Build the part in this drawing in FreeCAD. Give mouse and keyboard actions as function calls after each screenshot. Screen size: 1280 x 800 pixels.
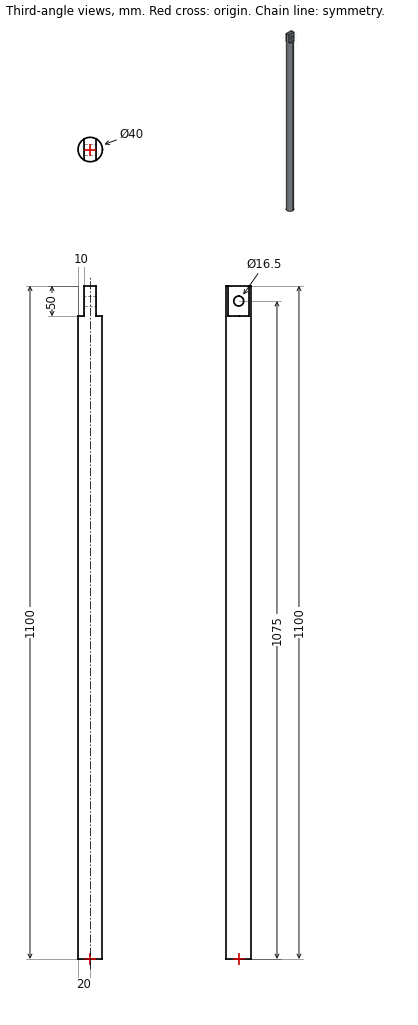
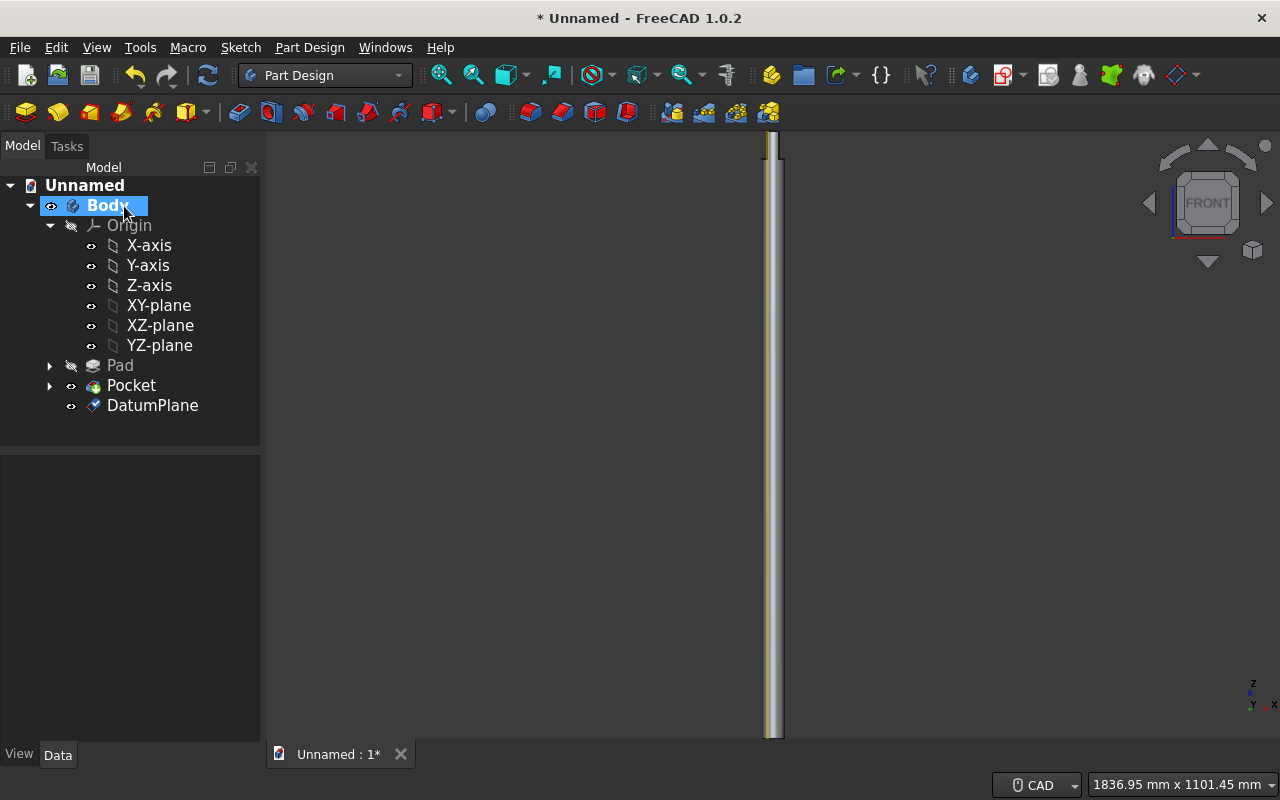
click(116, 406)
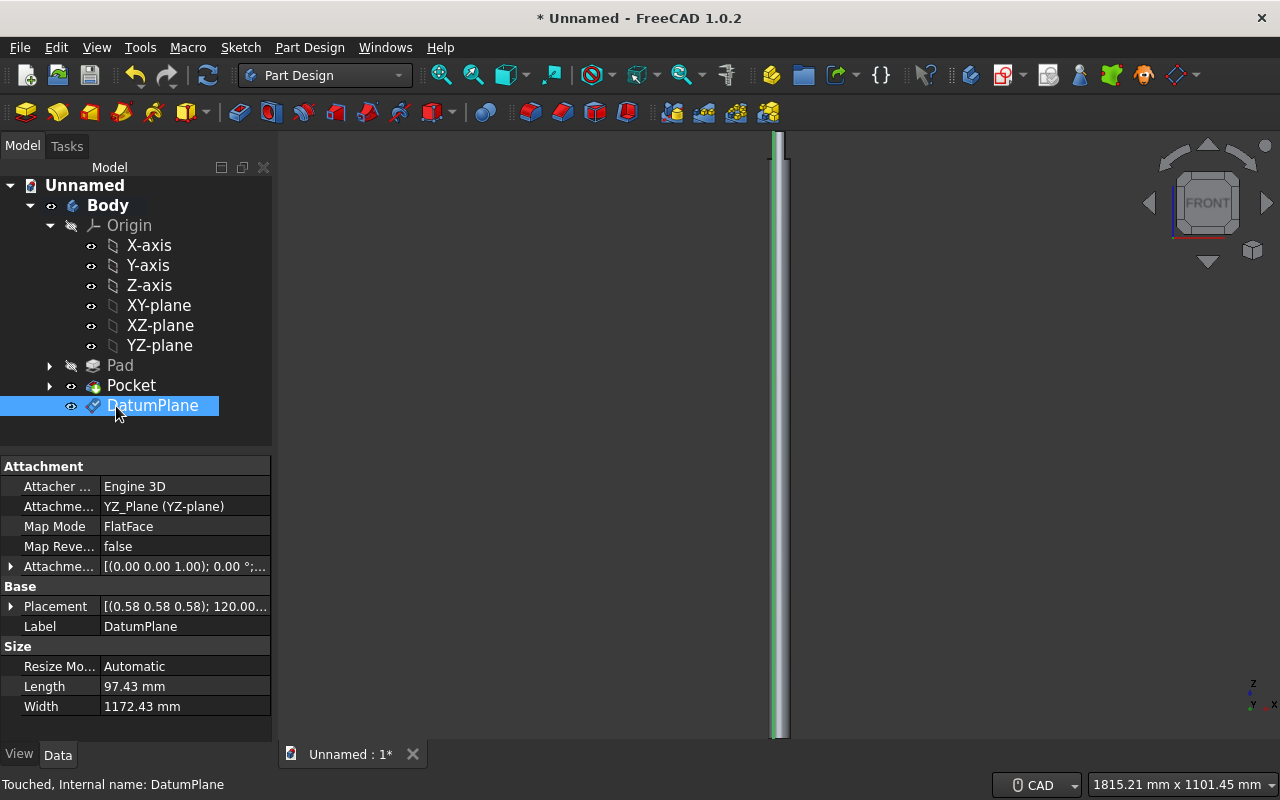
click(1004, 76)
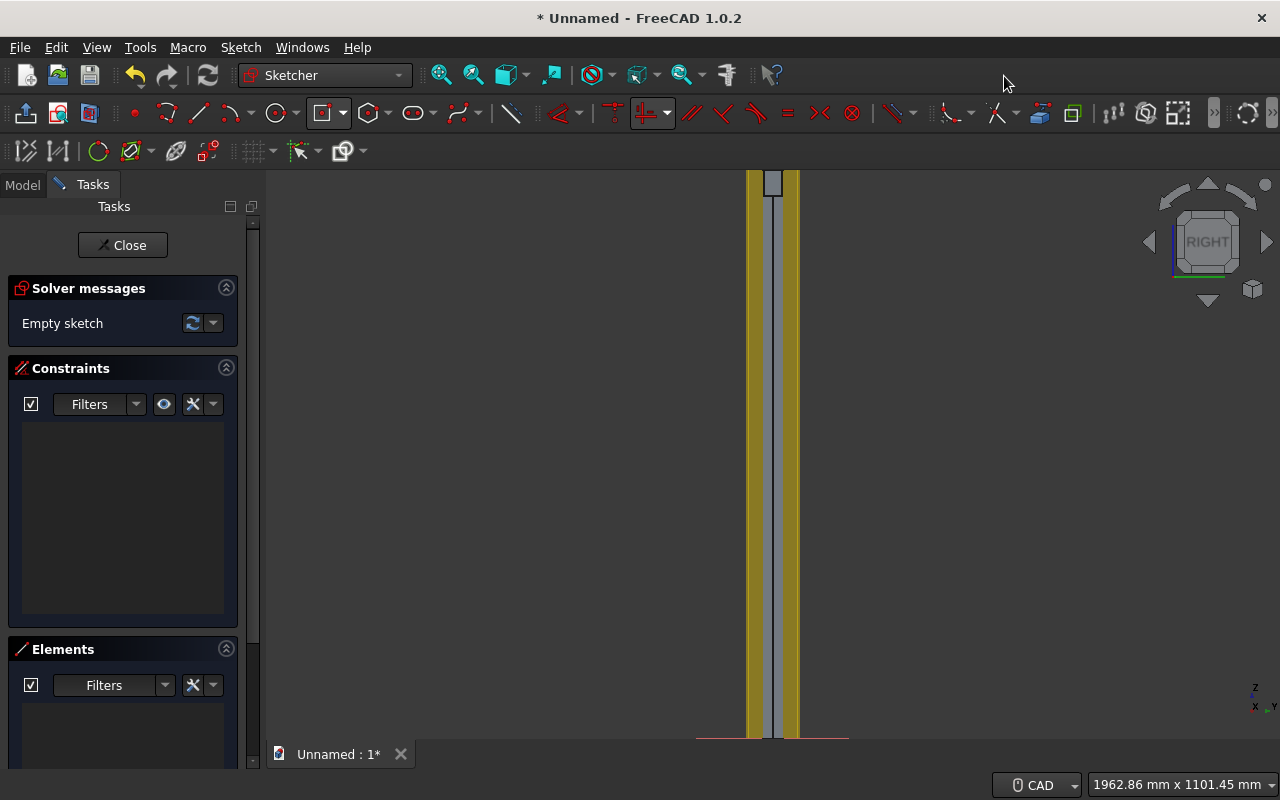
click(90, 114)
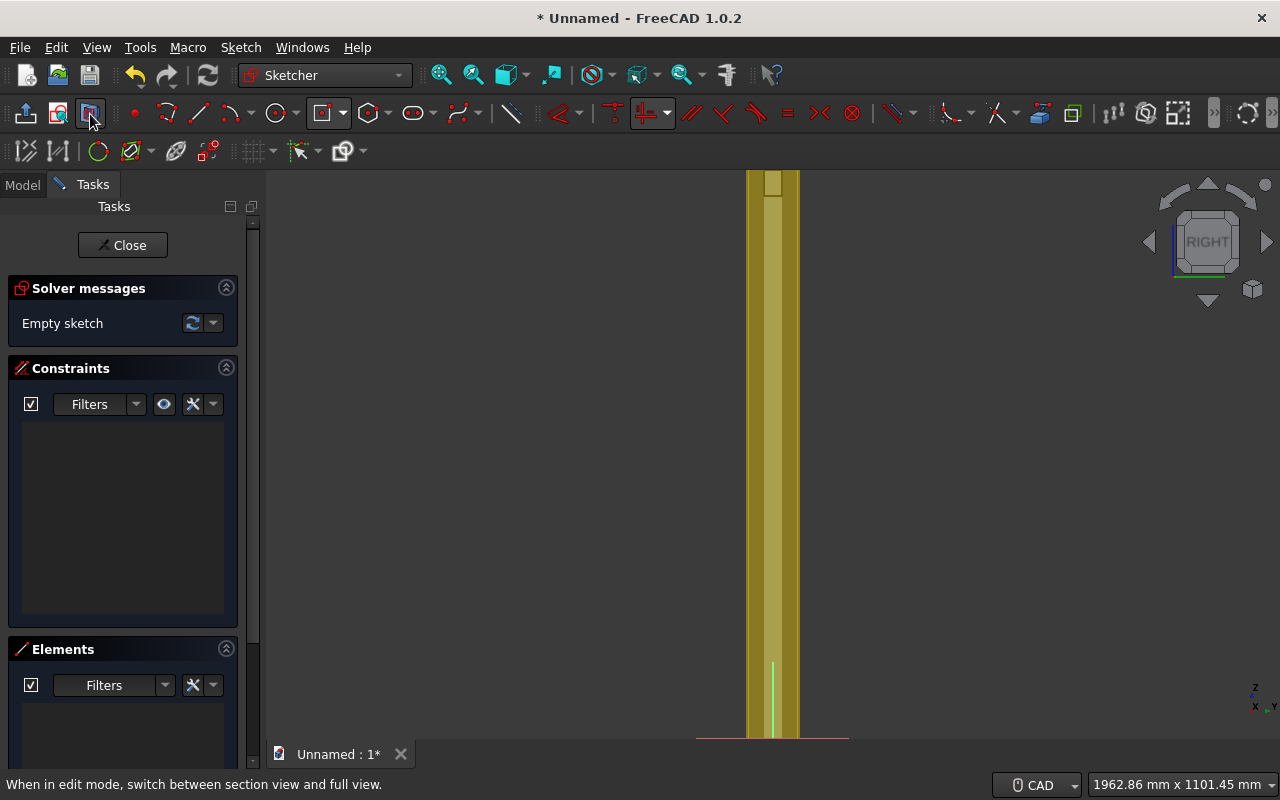
scroll(704, 454, down, 5)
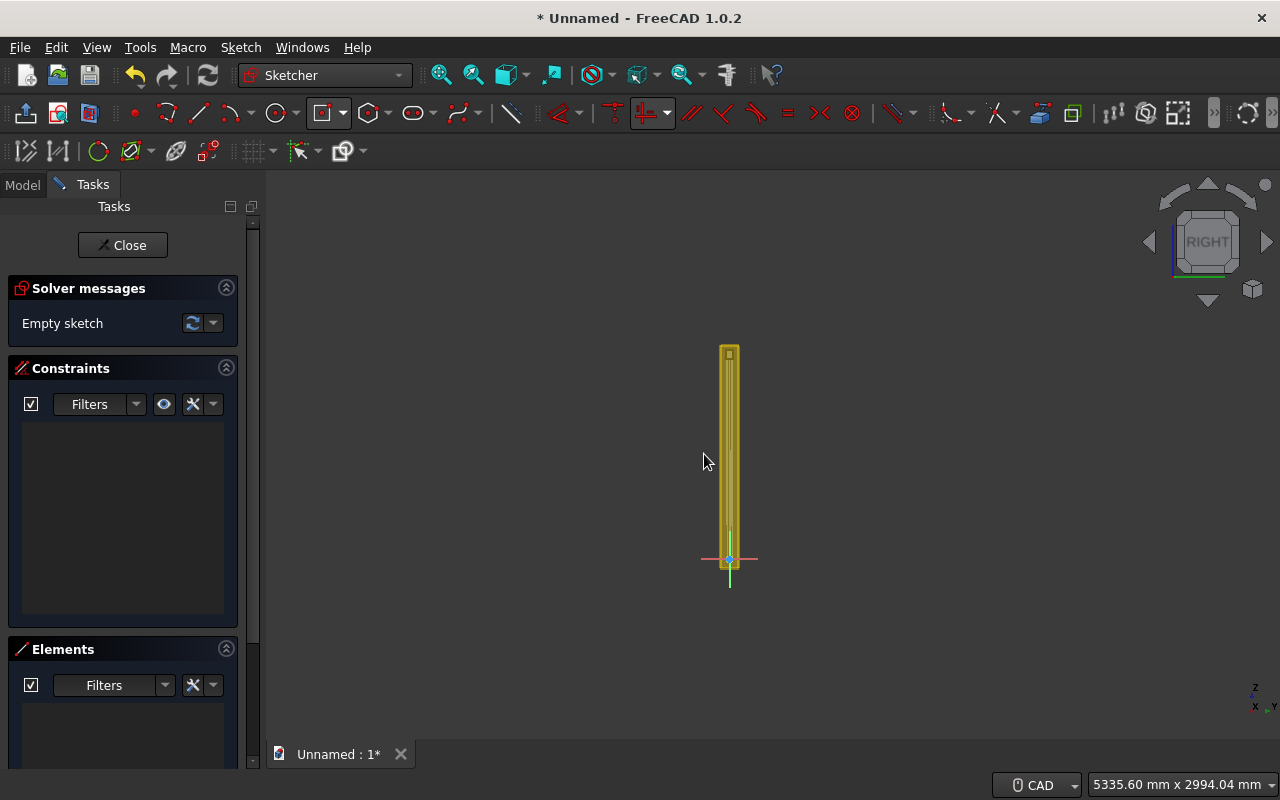
scroll(731, 349, up, 15)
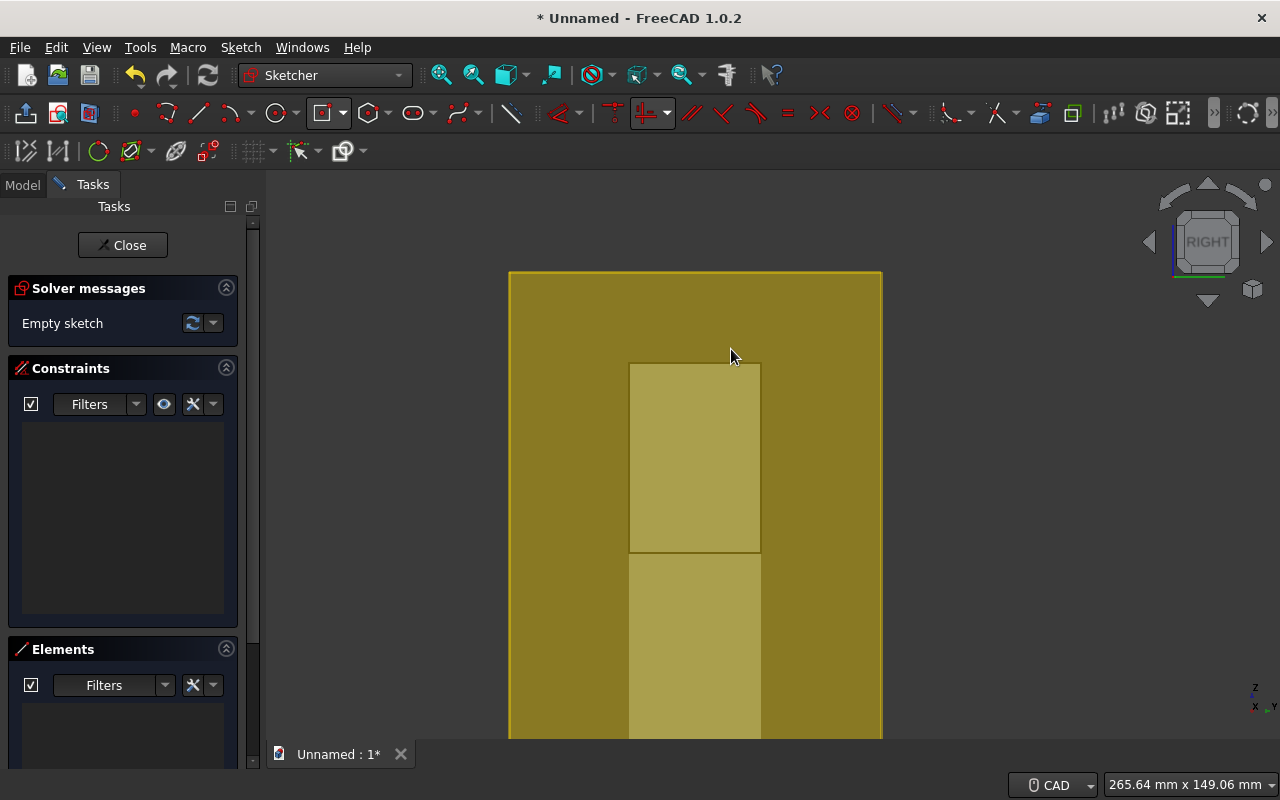
scroll(693, 459, up, 9)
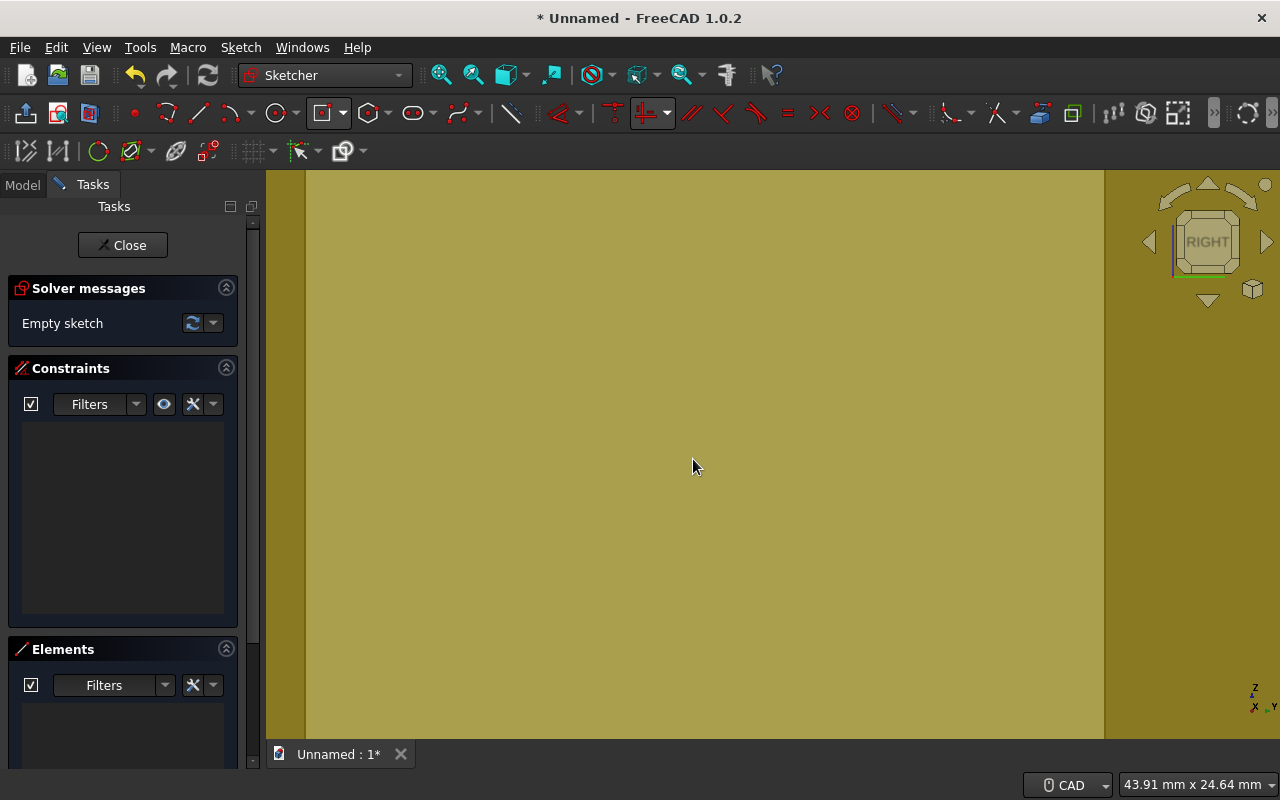
click(276, 114)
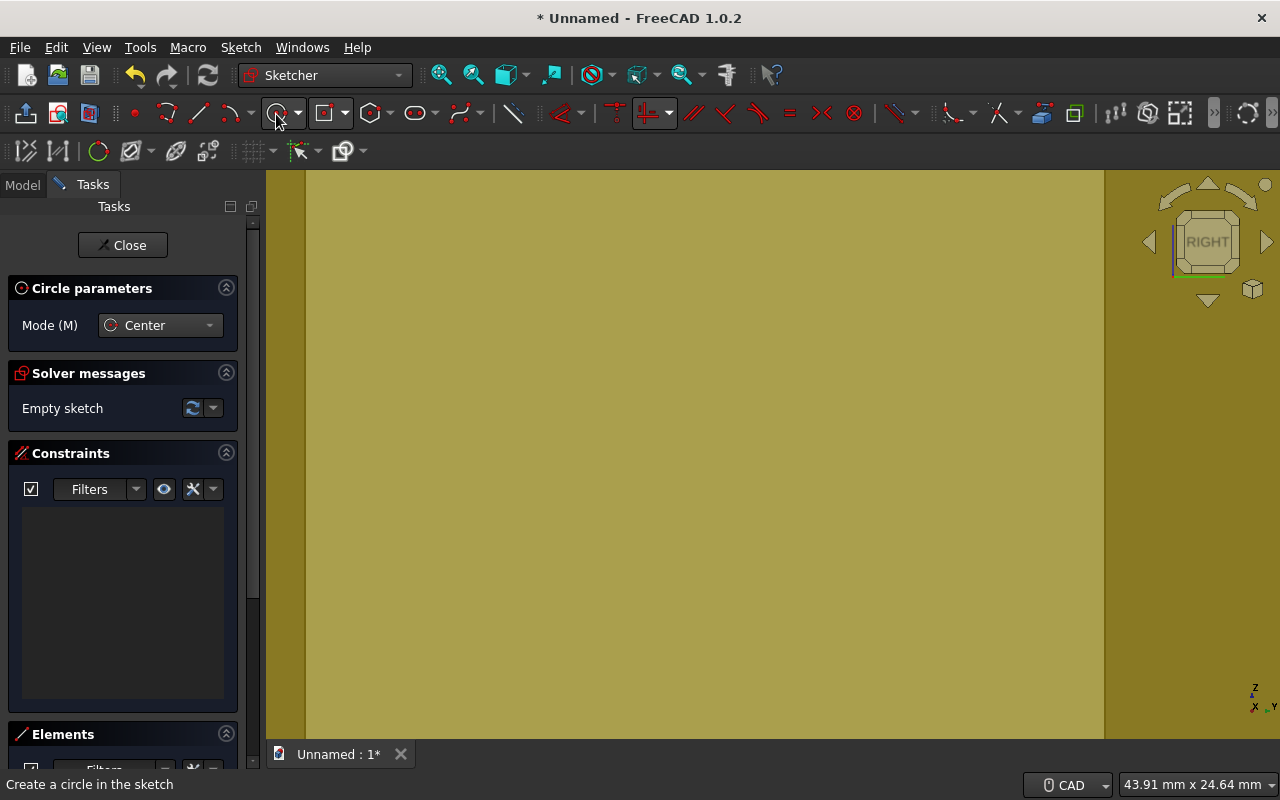
click(705, 450)
click(839, 316)
key(Escape)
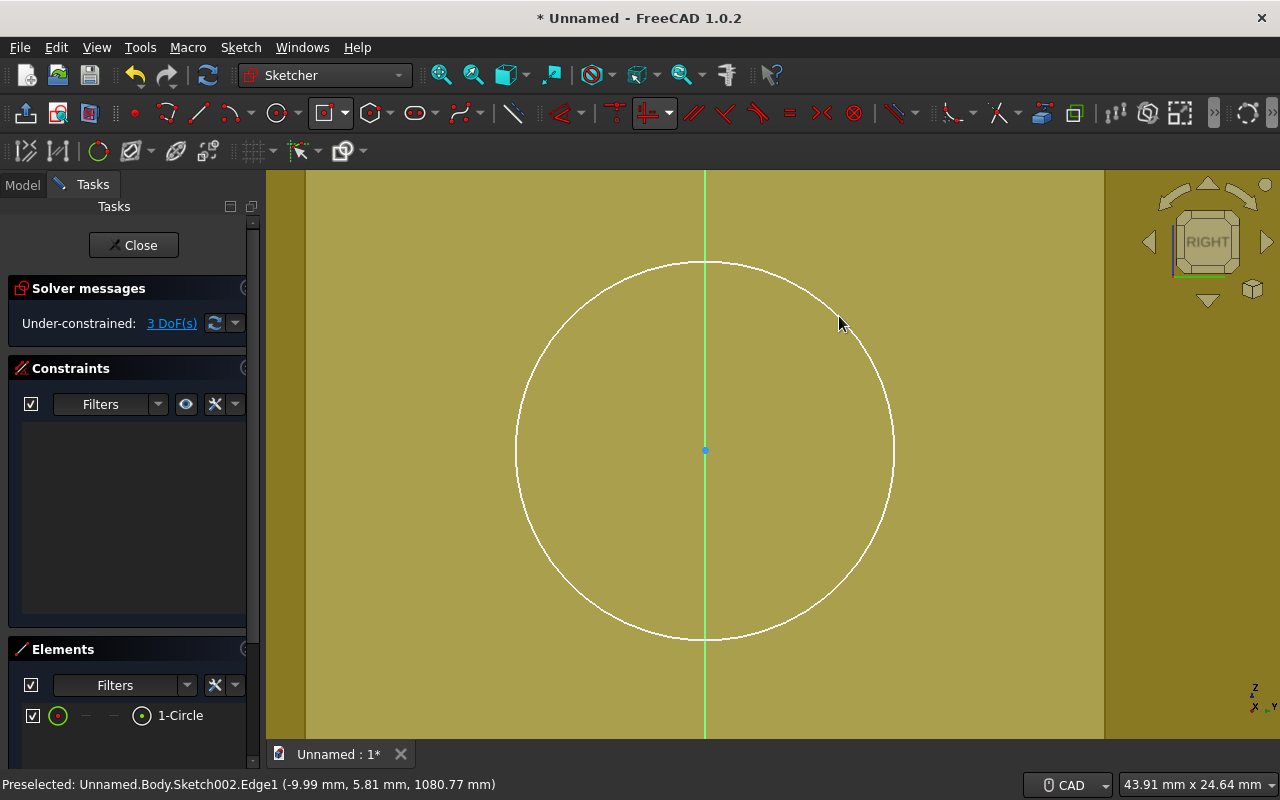
click(705, 451)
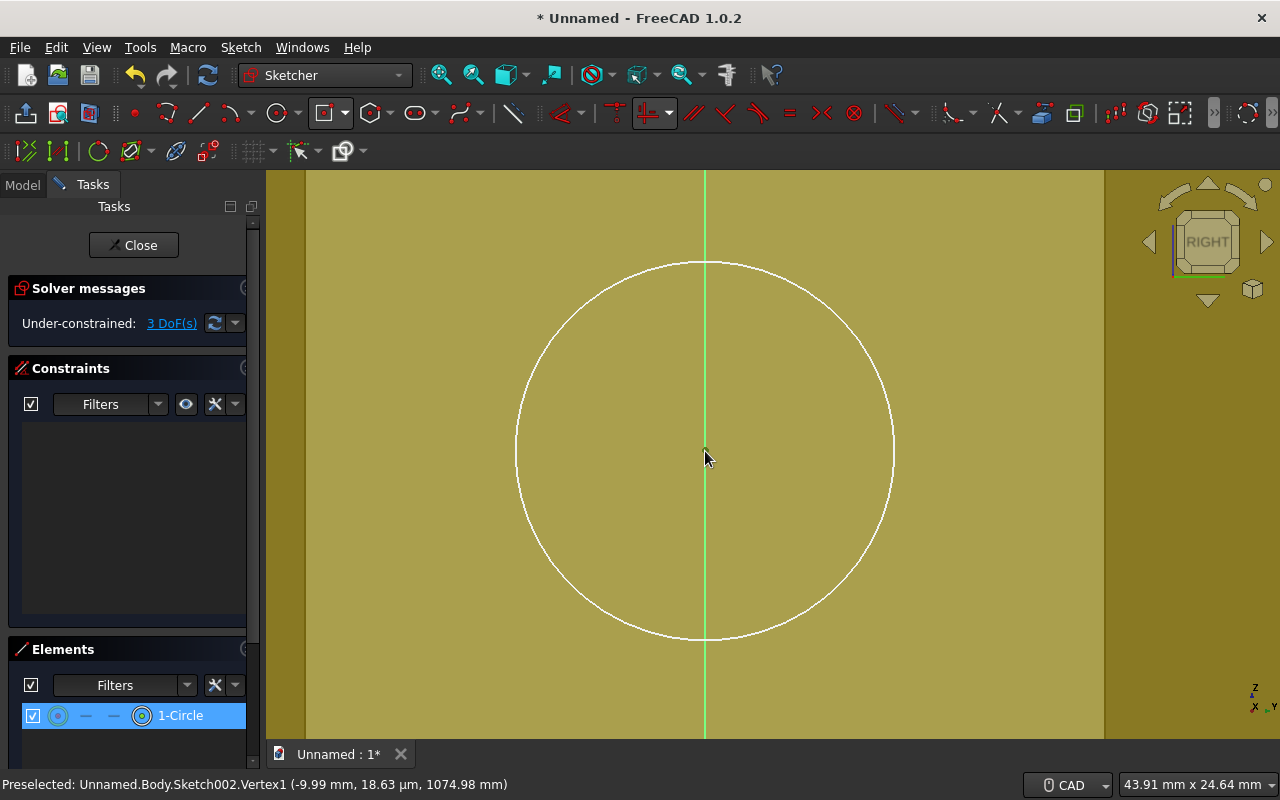
click(705, 674)